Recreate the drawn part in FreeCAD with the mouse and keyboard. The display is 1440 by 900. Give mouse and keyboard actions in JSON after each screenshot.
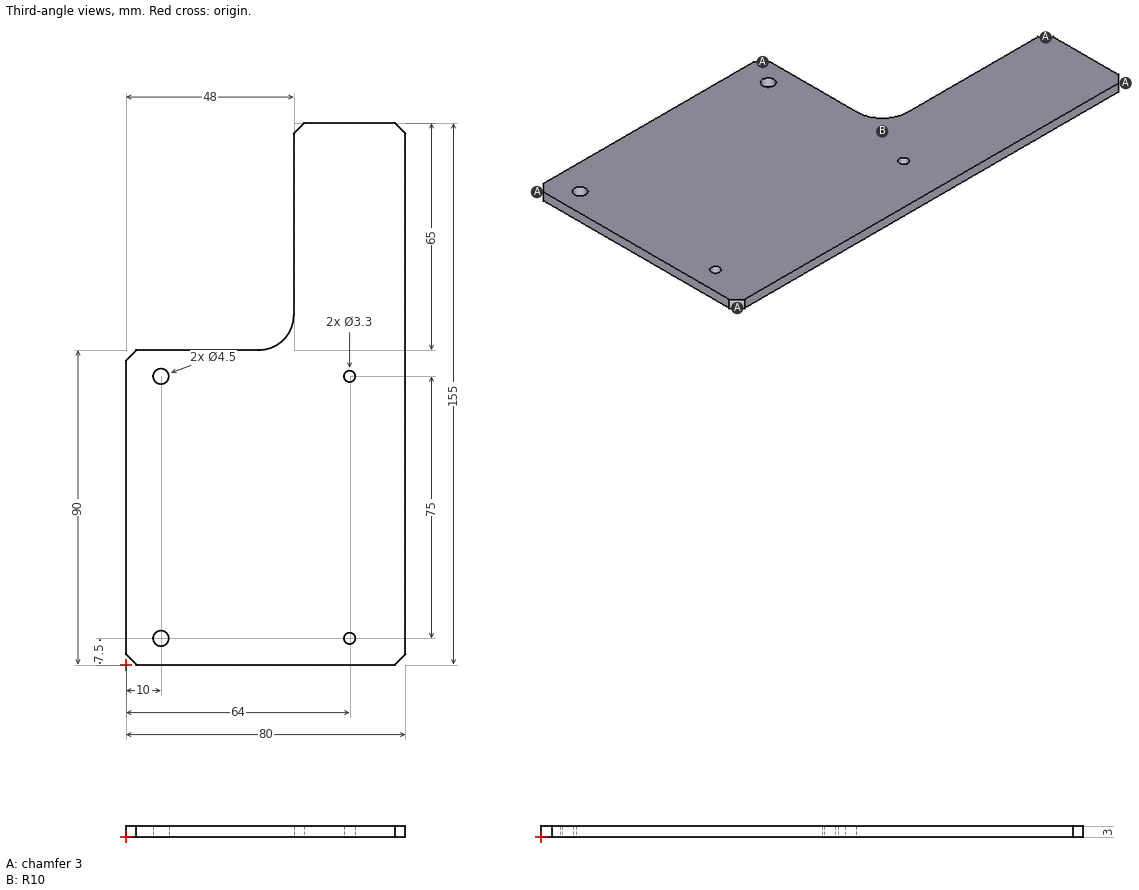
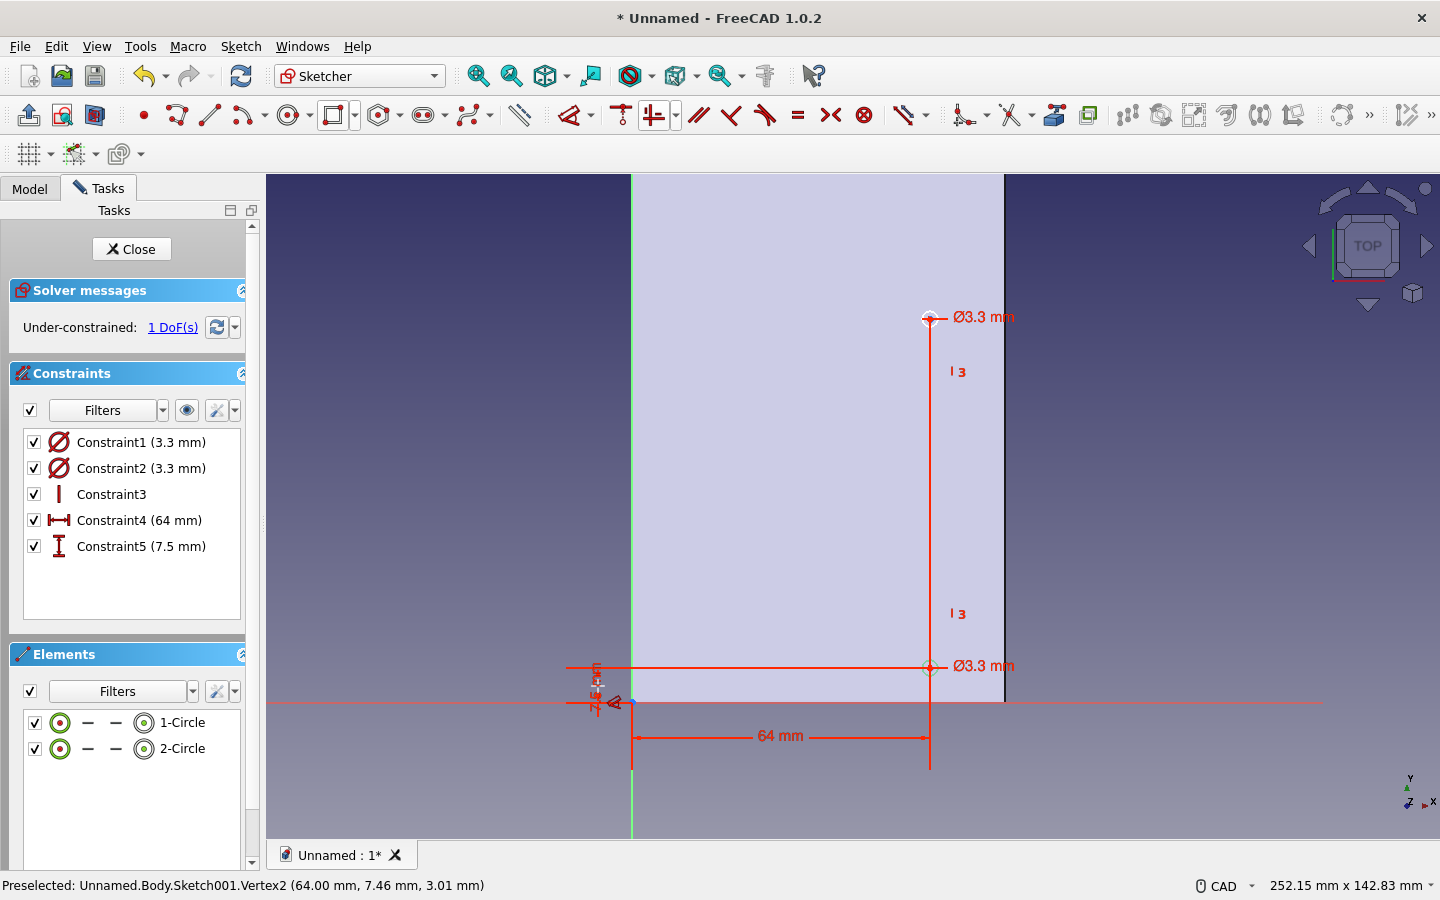
{"action": "left_click", "coordinate": [930, 319]}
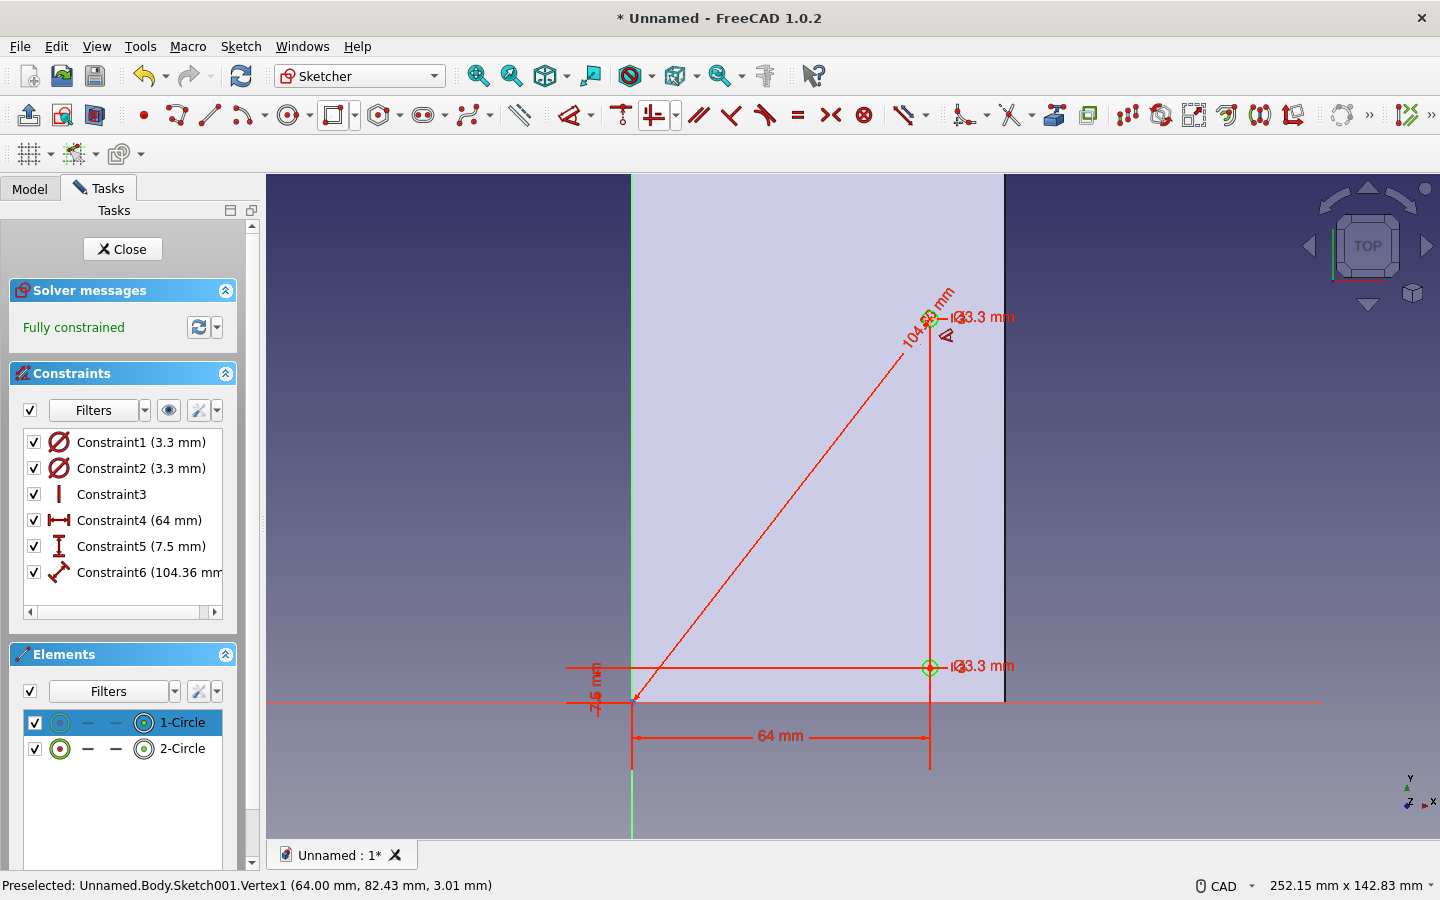
{"action": "left_click", "coordinate": [930, 668]}
{"action": "left_click", "coordinate": [964, 494]}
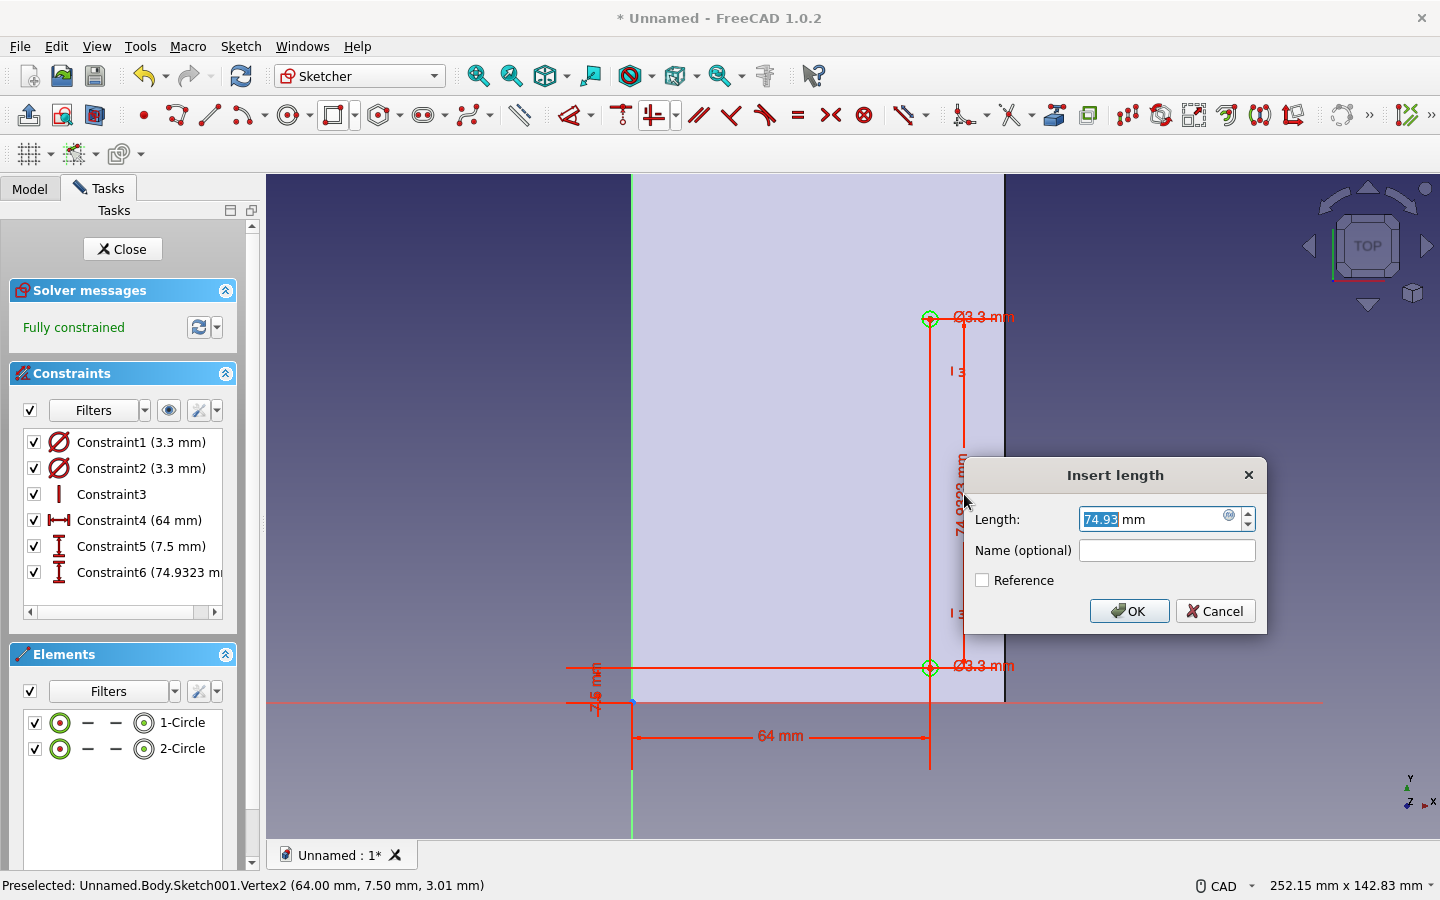
{"action": "type", "text": "75"}
{"action": "key", "text": "Return"}
{"action": "key", "text": "Escape"}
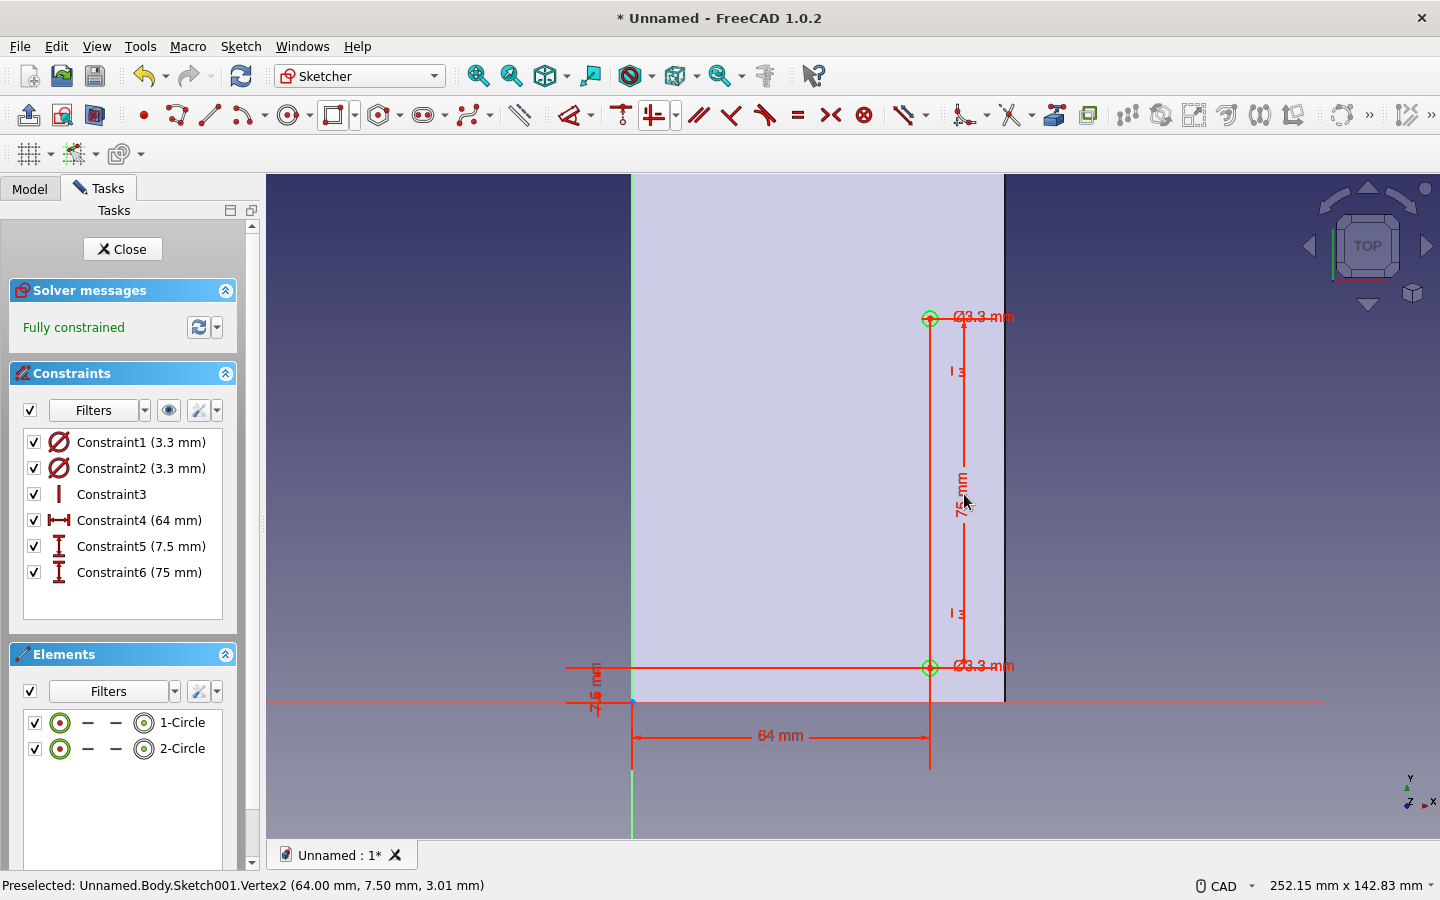
{"action": "left_click", "coordinate": [123, 249]}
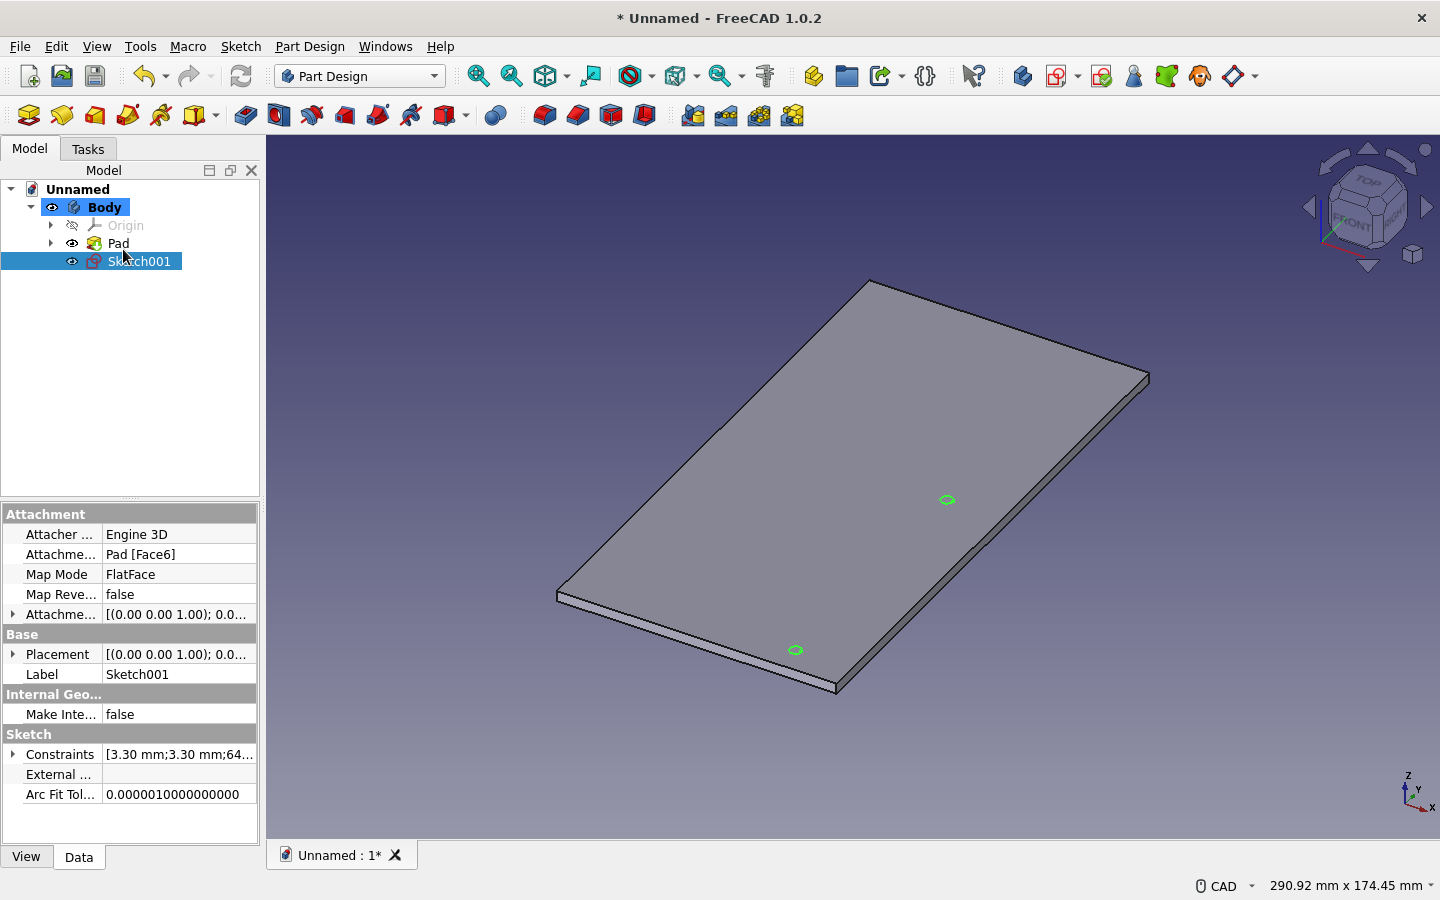
{"action": "left_click", "coordinate": [246, 116]}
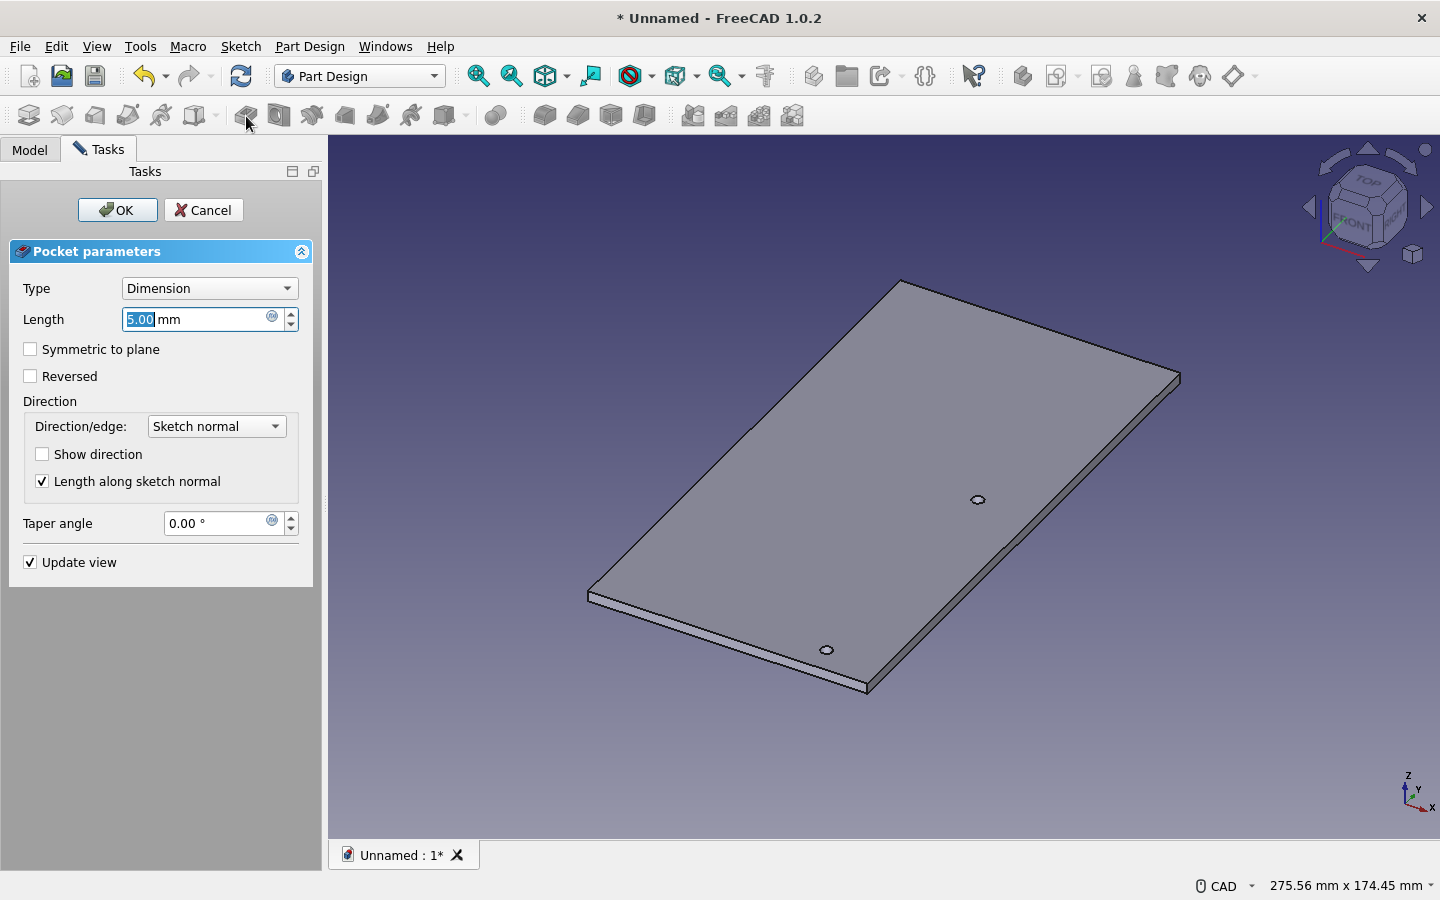
{"action": "left_click", "coordinate": [210, 288]}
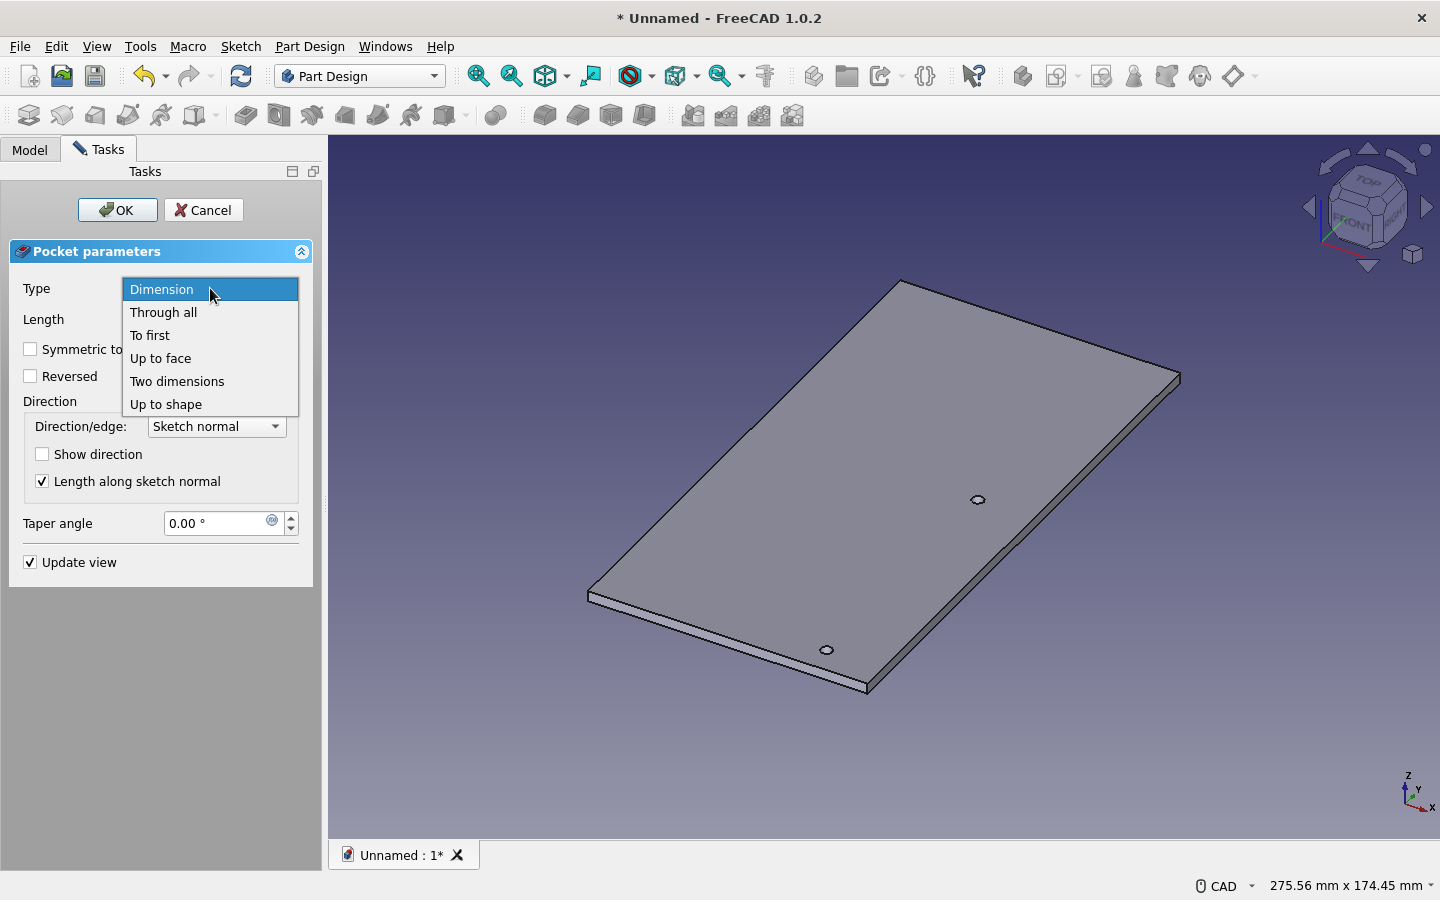
{"action": "left_click", "coordinate": [208, 312]}